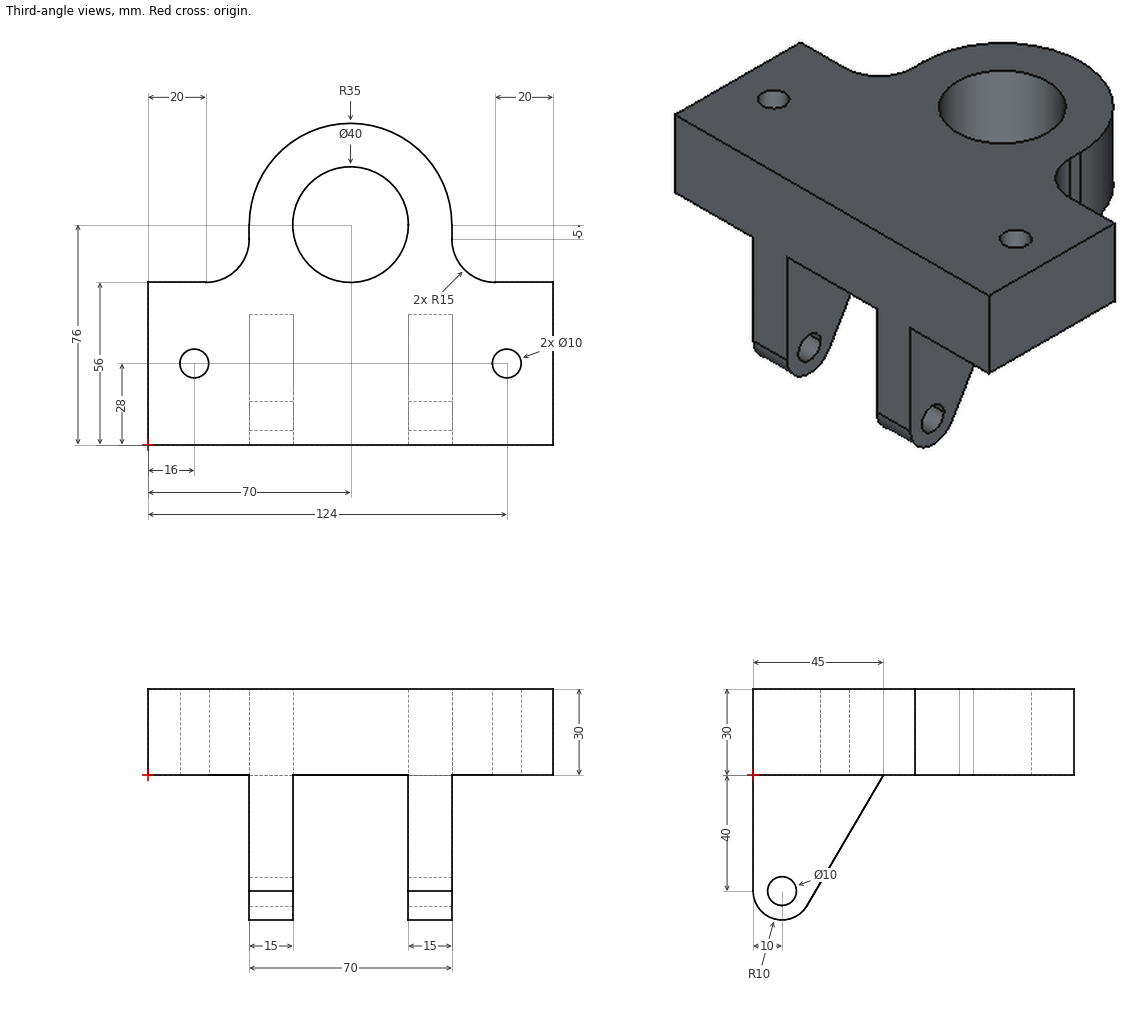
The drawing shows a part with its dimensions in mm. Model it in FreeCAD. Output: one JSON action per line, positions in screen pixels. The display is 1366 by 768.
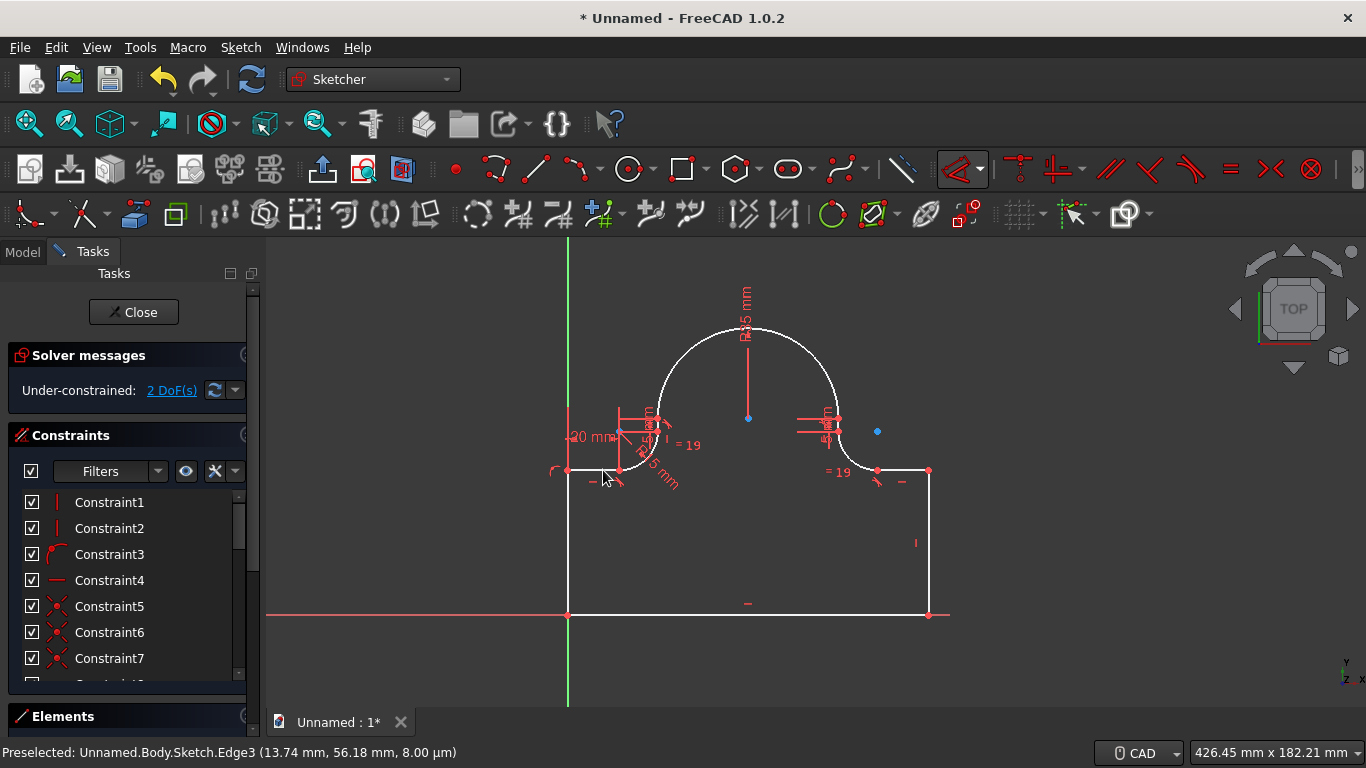
{"action": "left_click", "coordinate": [568, 514]}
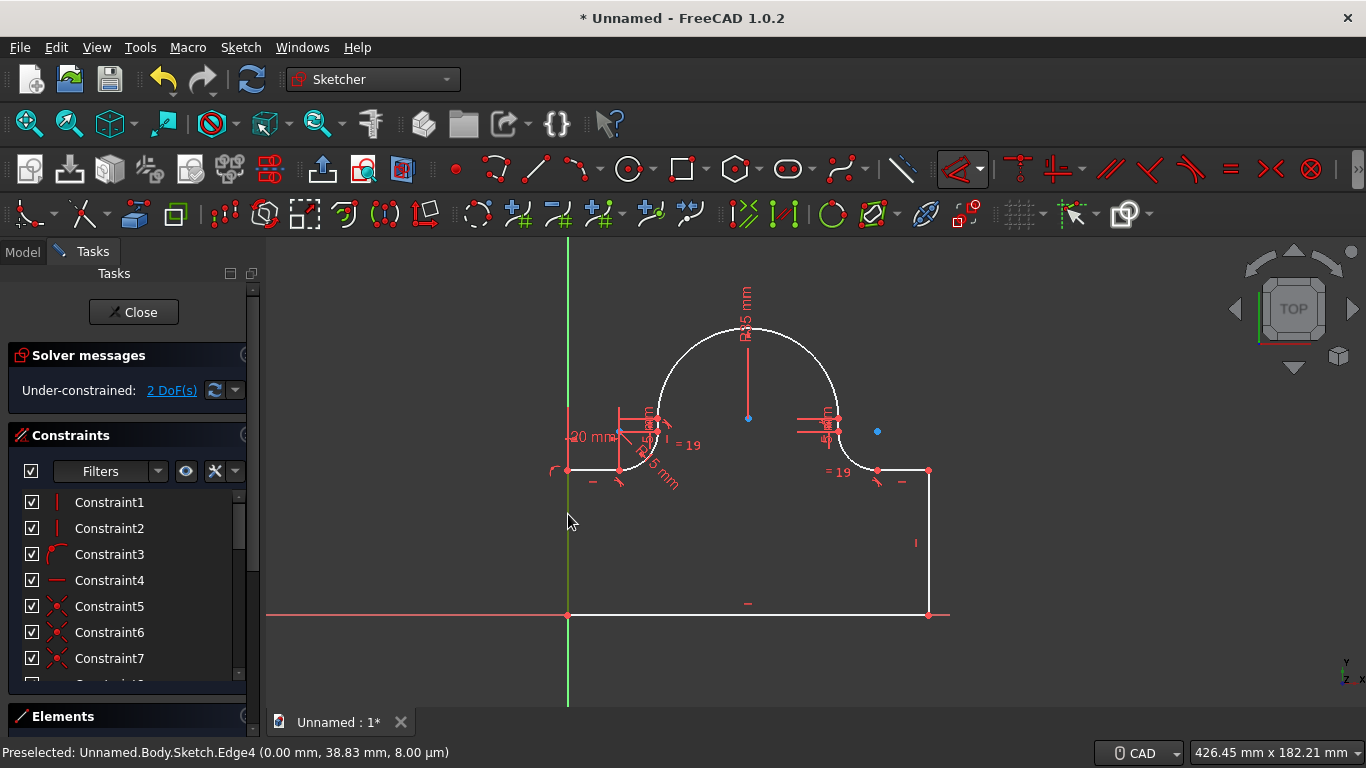
{"action": "key", "text": "i"}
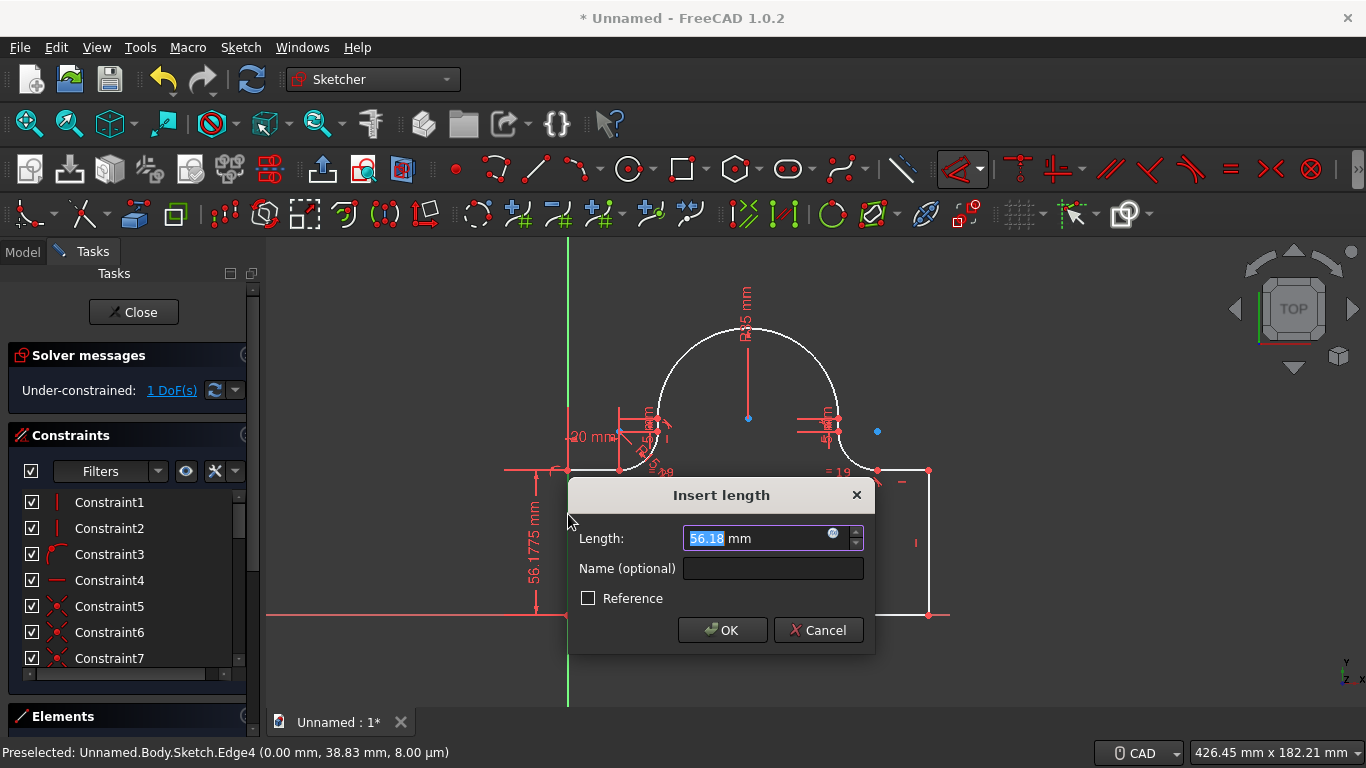
{"action": "type", "text": "56"}
{"action": "key", "text": "Return"}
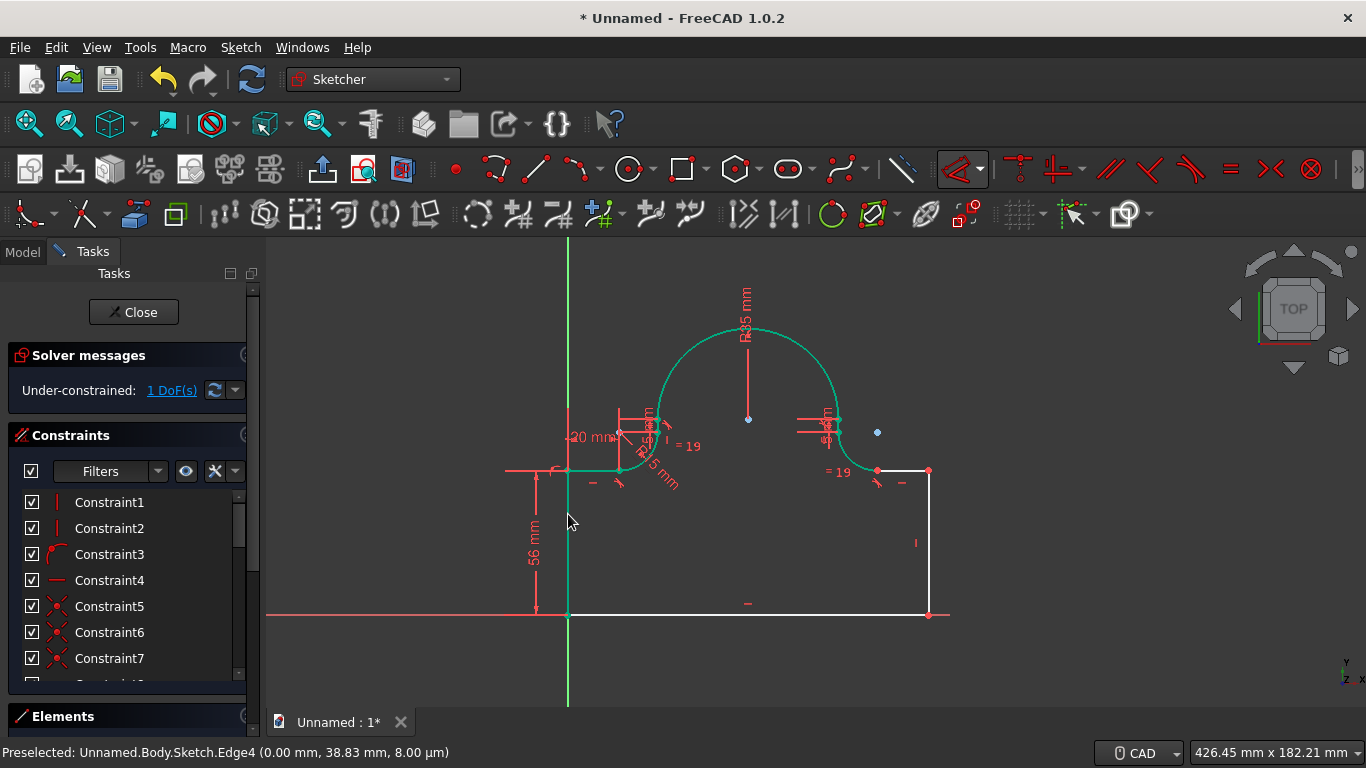
{"action": "left_click", "coordinate": [913, 471]}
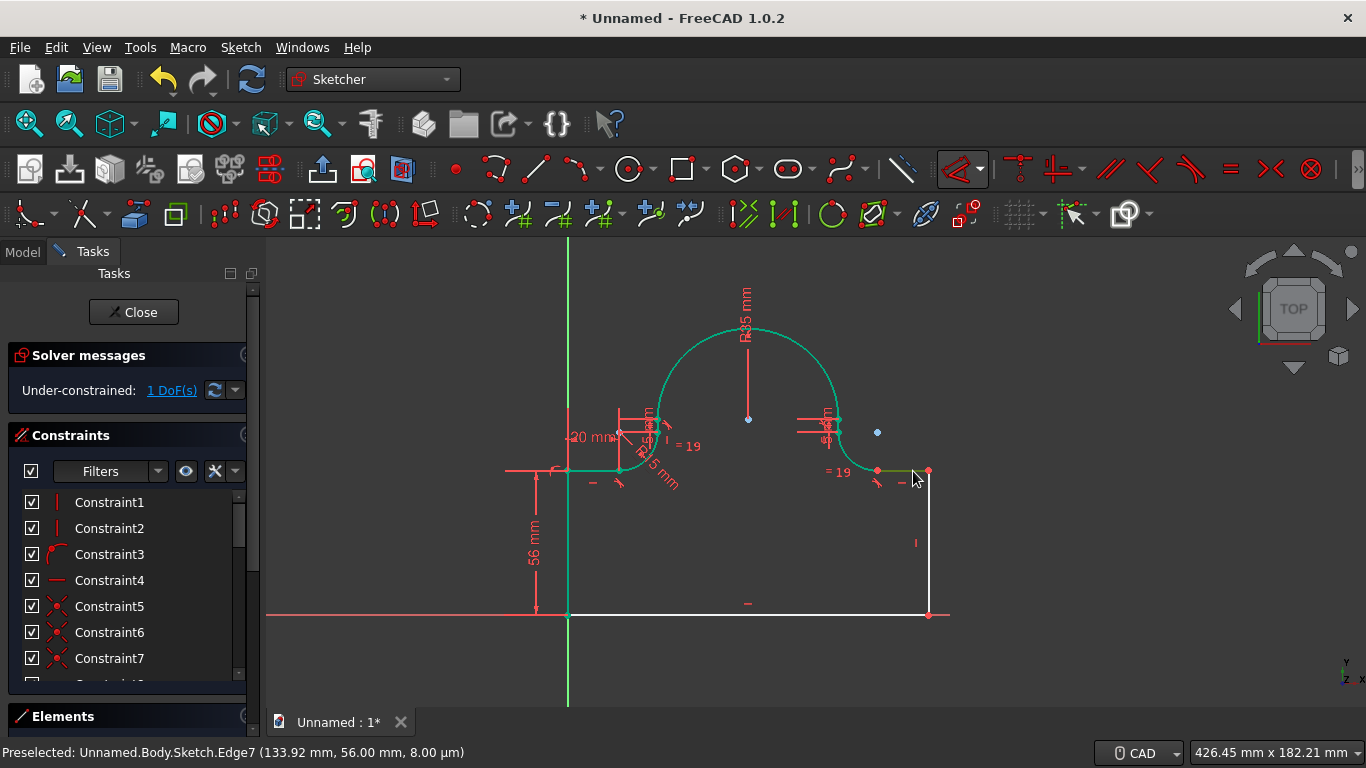
{"action": "left_click", "coordinate": [982, 170]}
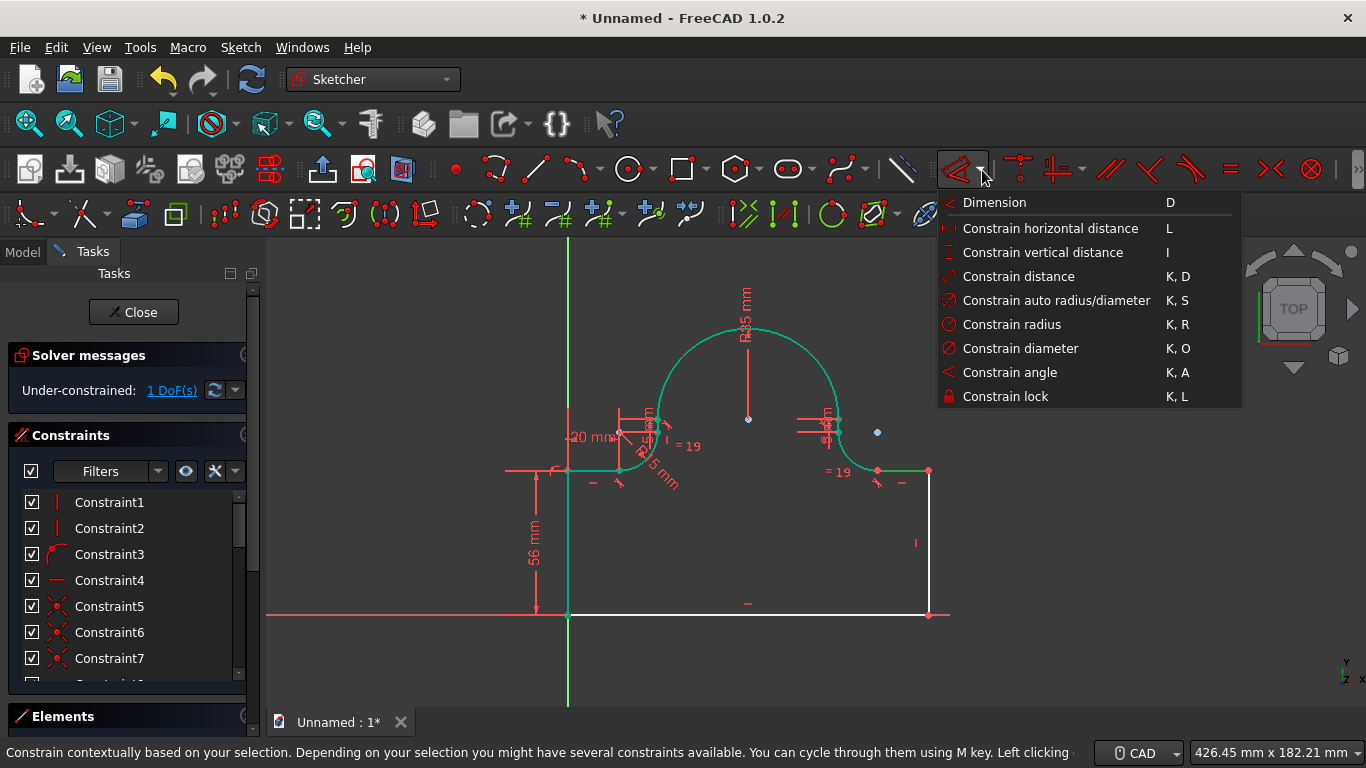
{"action": "left_click", "coordinate": [1090, 228]}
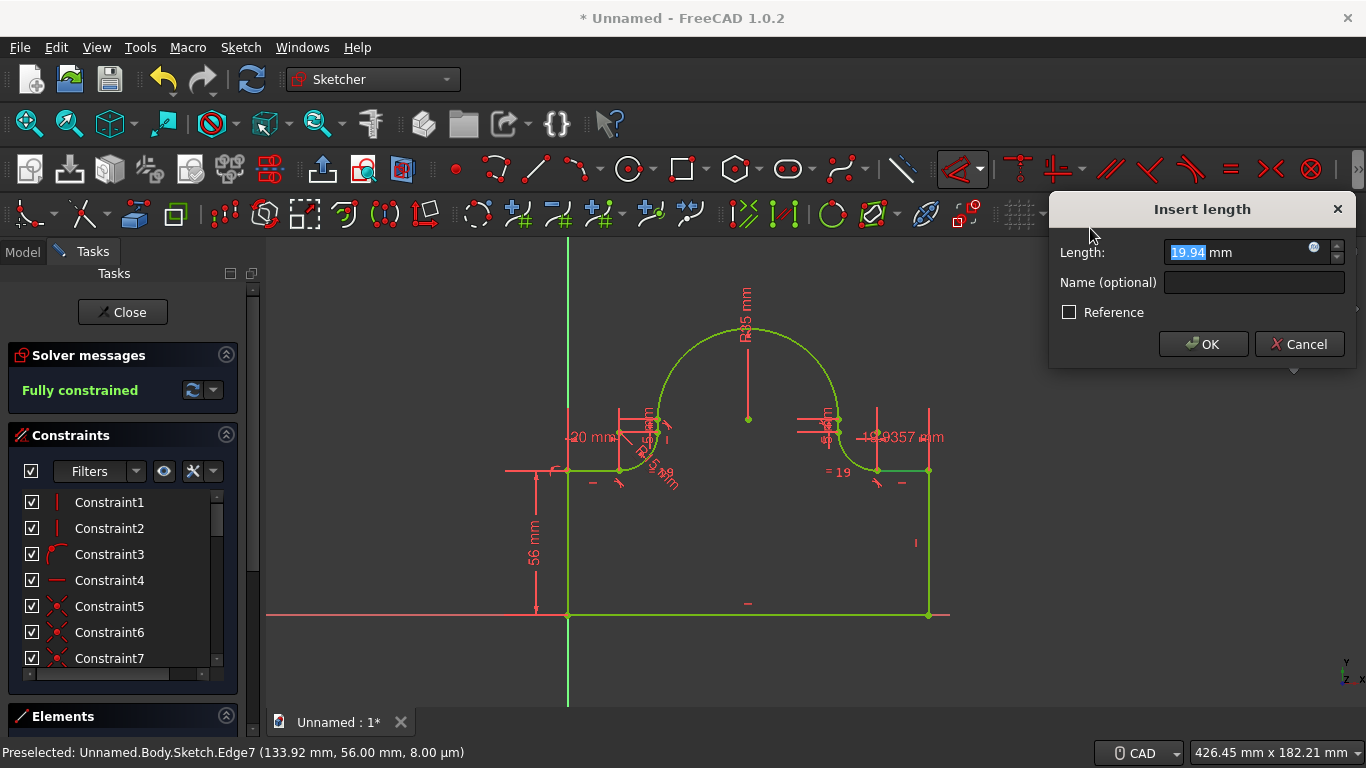
{"action": "type", "text": "20"}
{"action": "key", "text": "Return"}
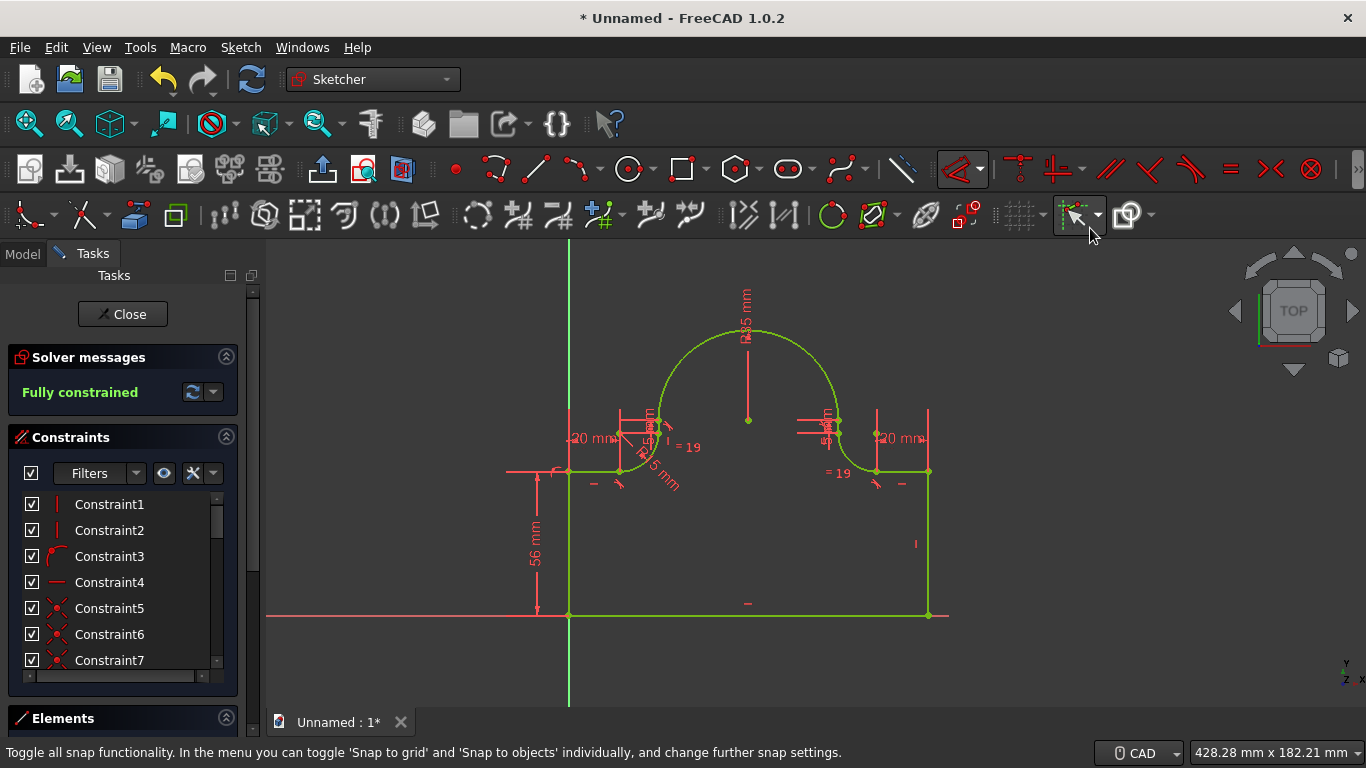
{"action": "left_click", "coordinate": [123, 314]}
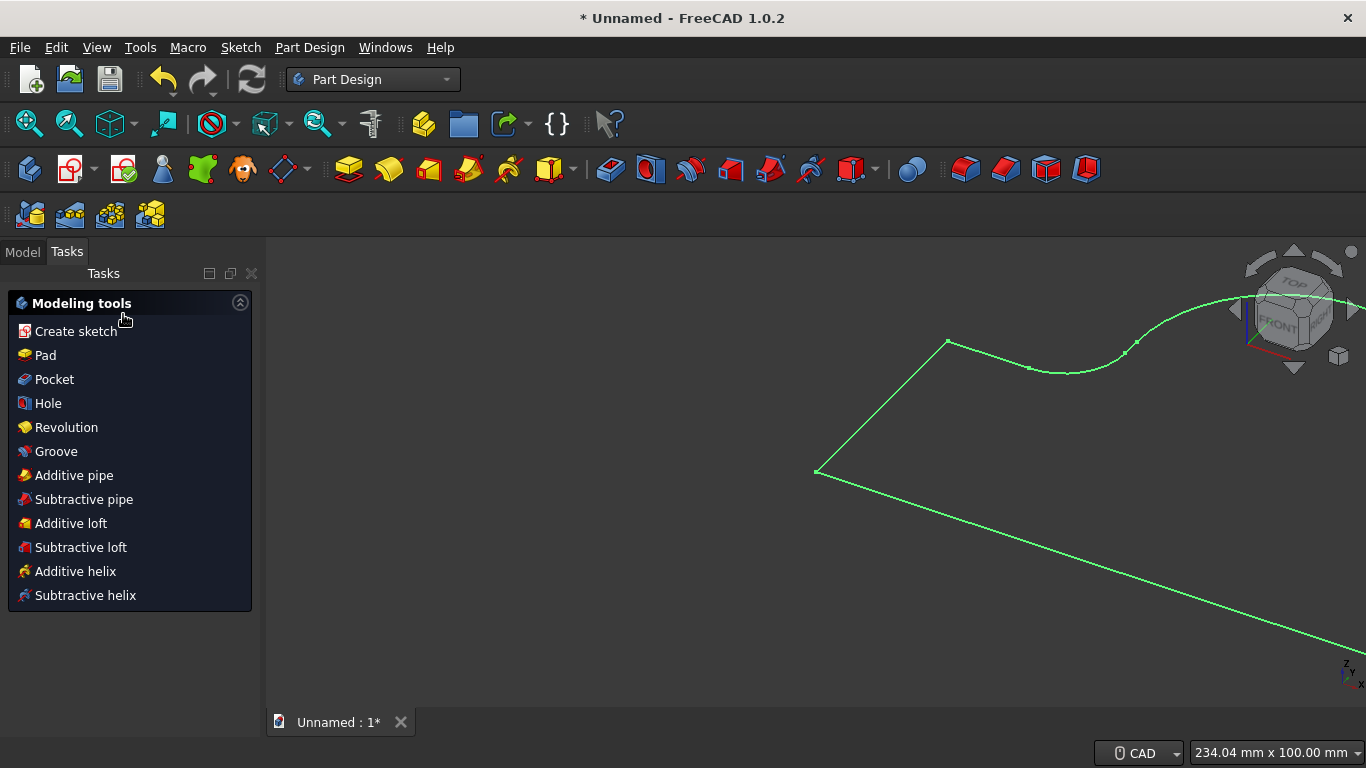
{"action": "left_click", "coordinate": [350, 170]}